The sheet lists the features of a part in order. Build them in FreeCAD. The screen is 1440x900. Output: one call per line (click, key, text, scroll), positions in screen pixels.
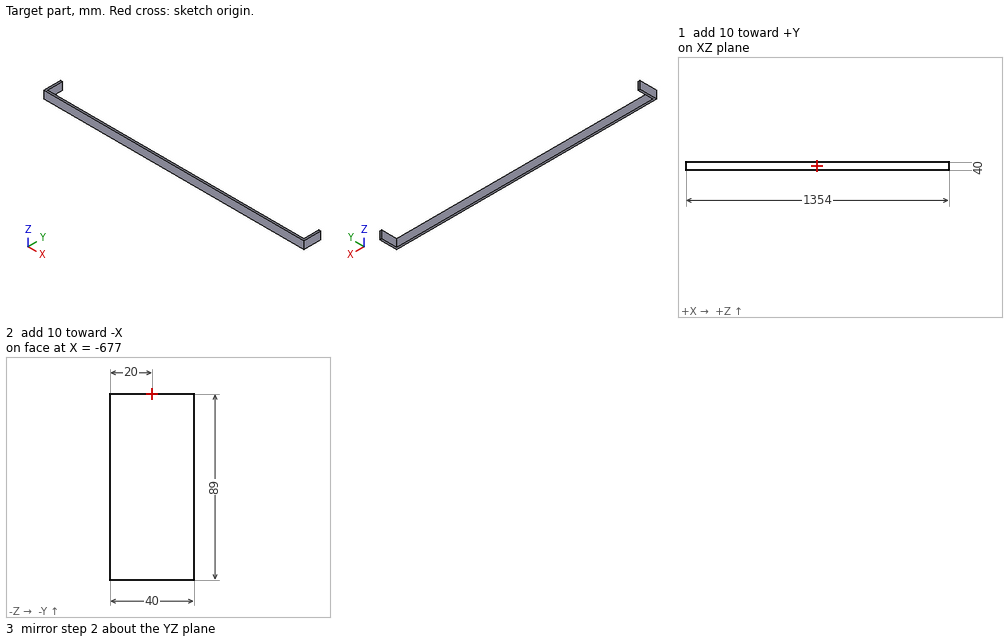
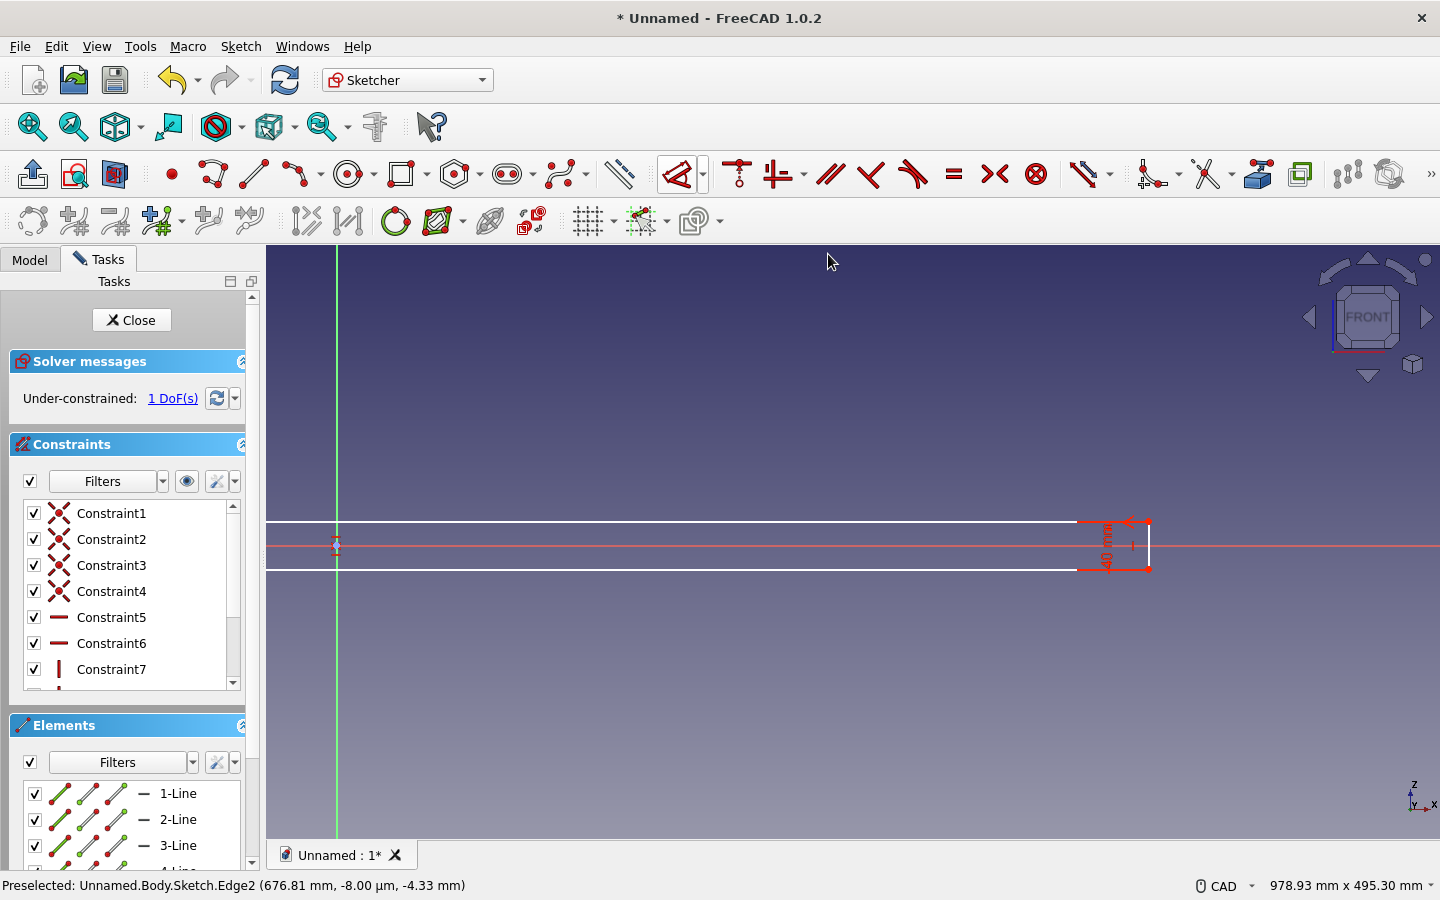
click(662, 570)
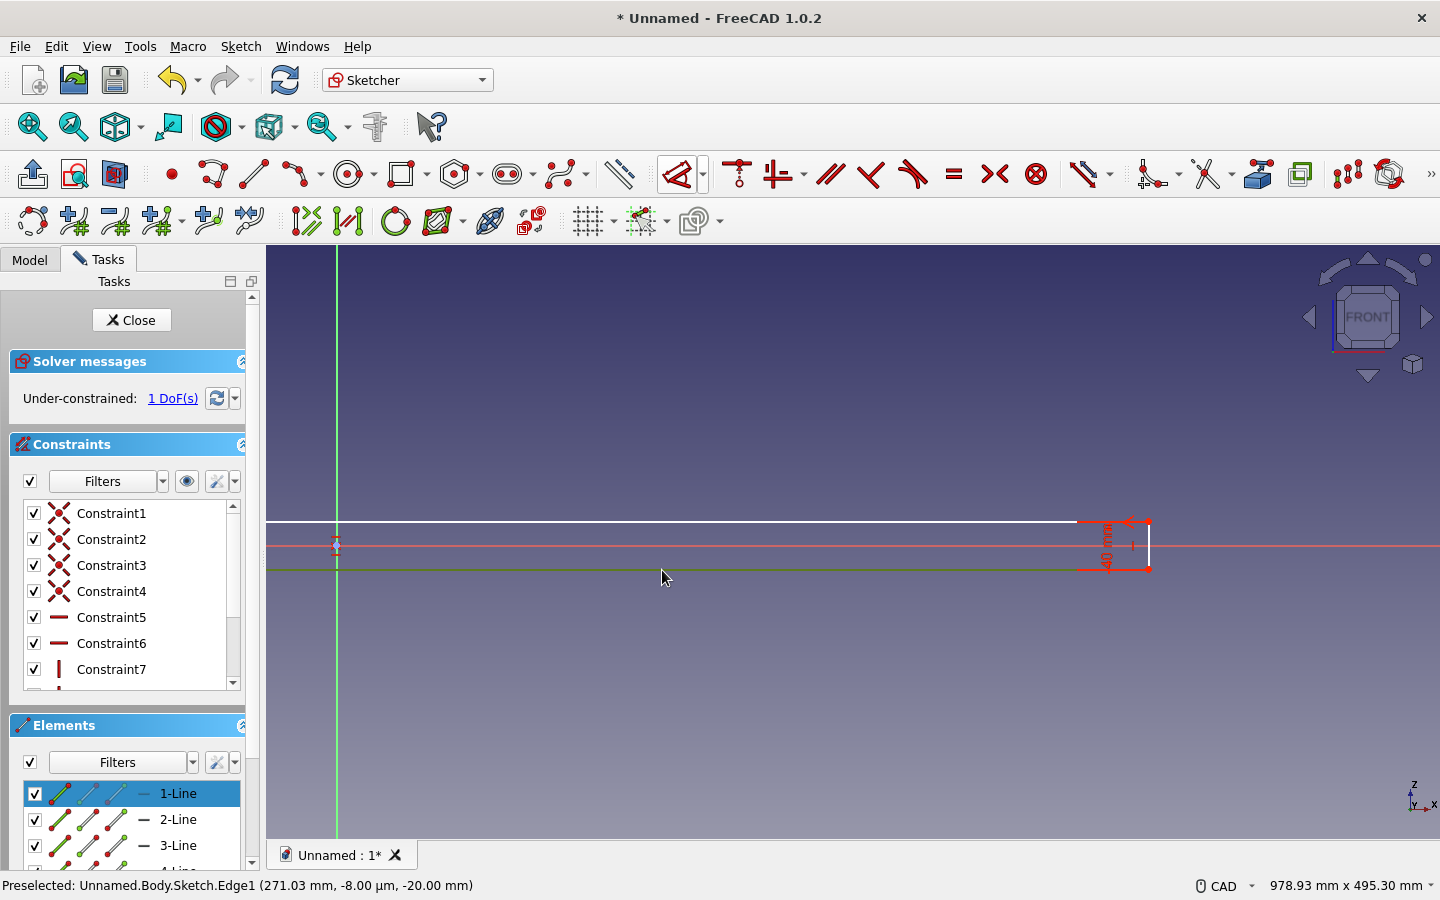
click(702, 174)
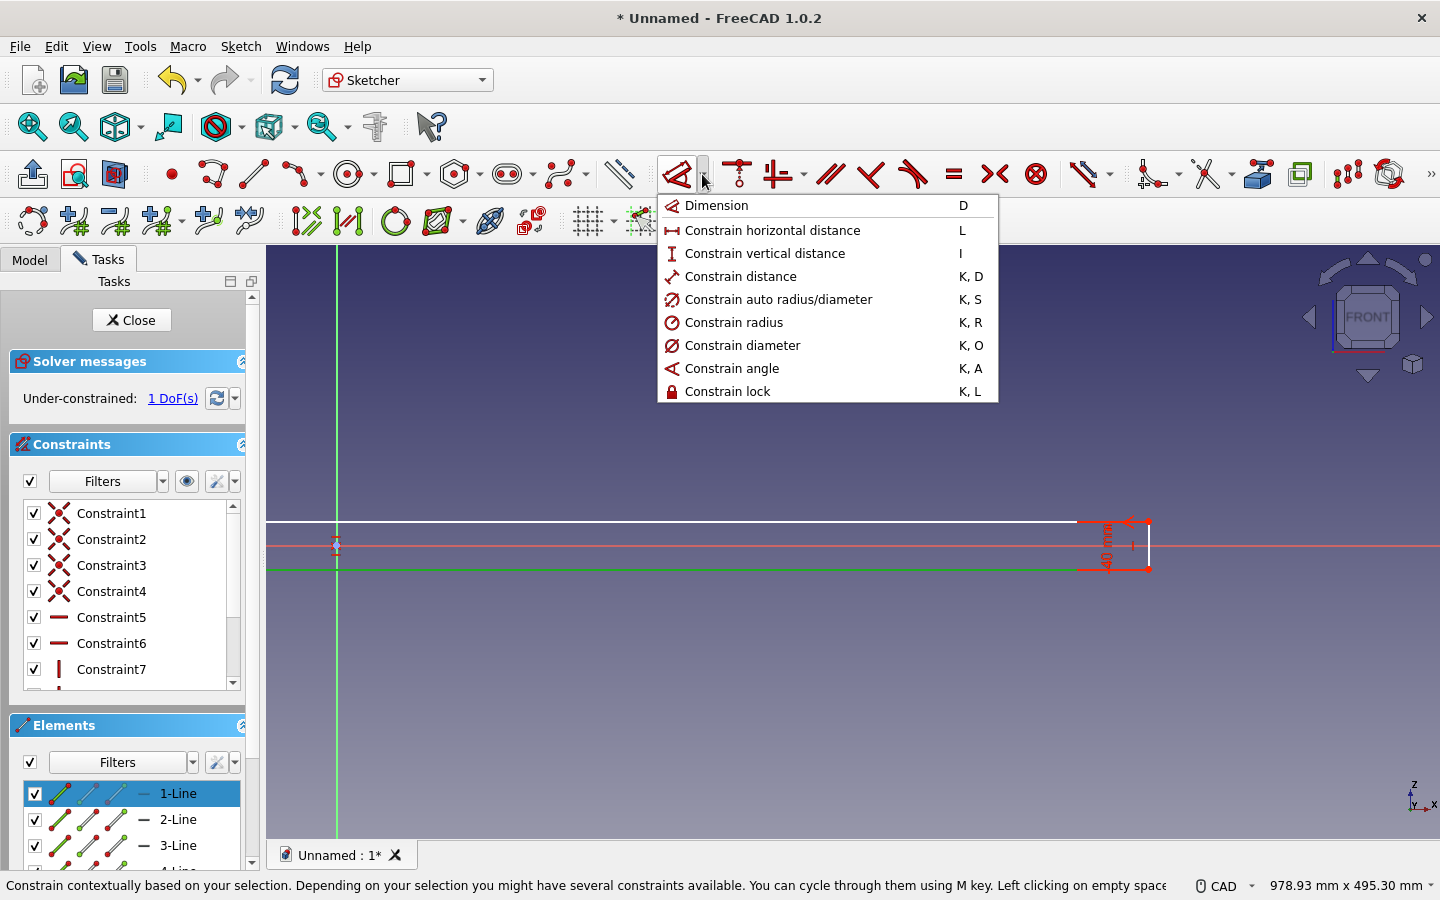
click(828, 230)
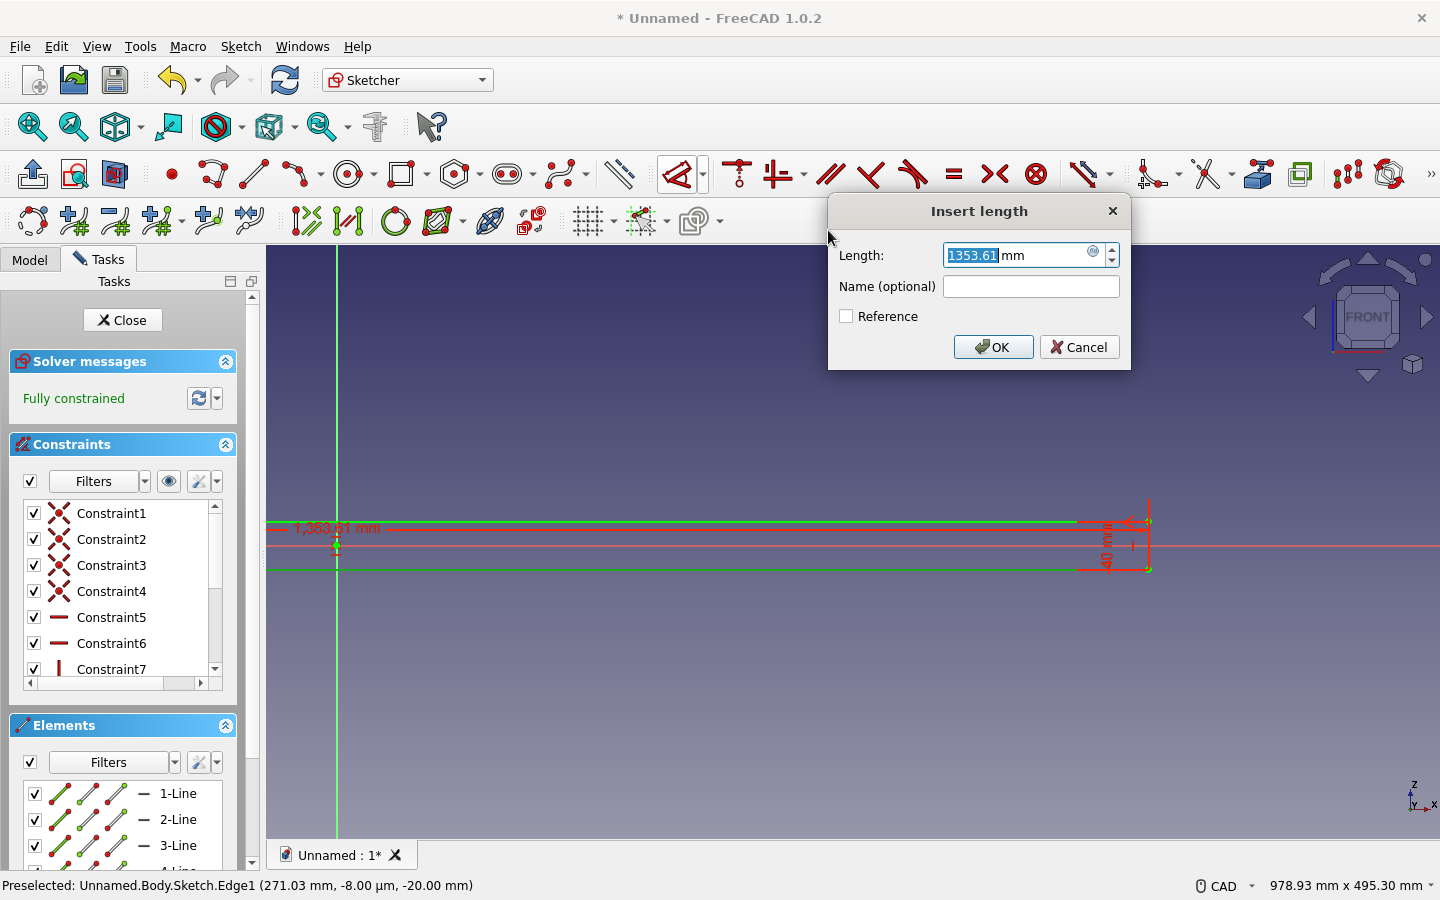
text(1354)
key(Return)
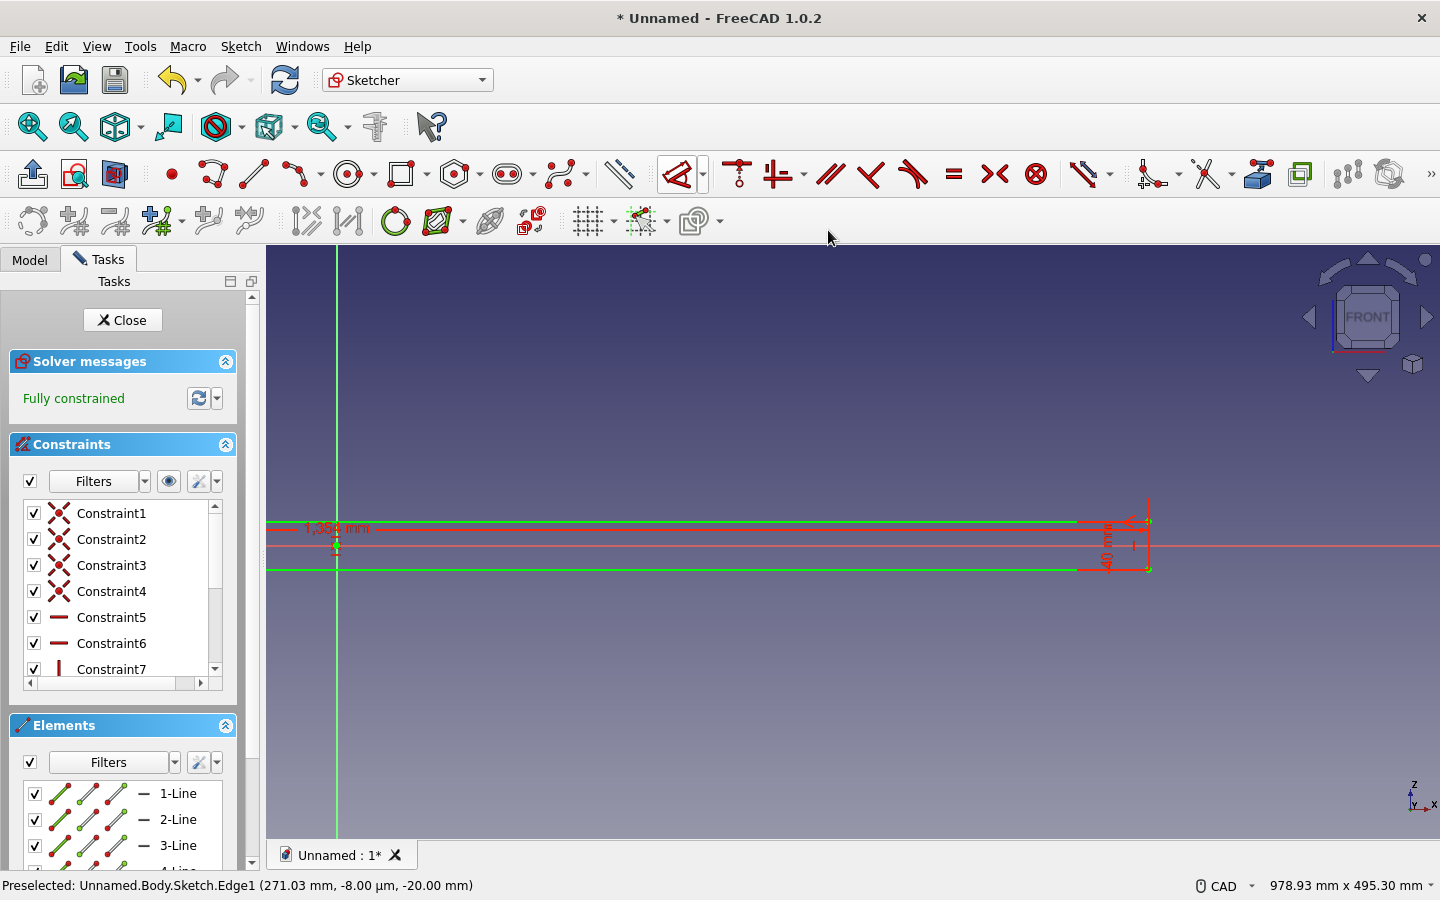
click(123, 320)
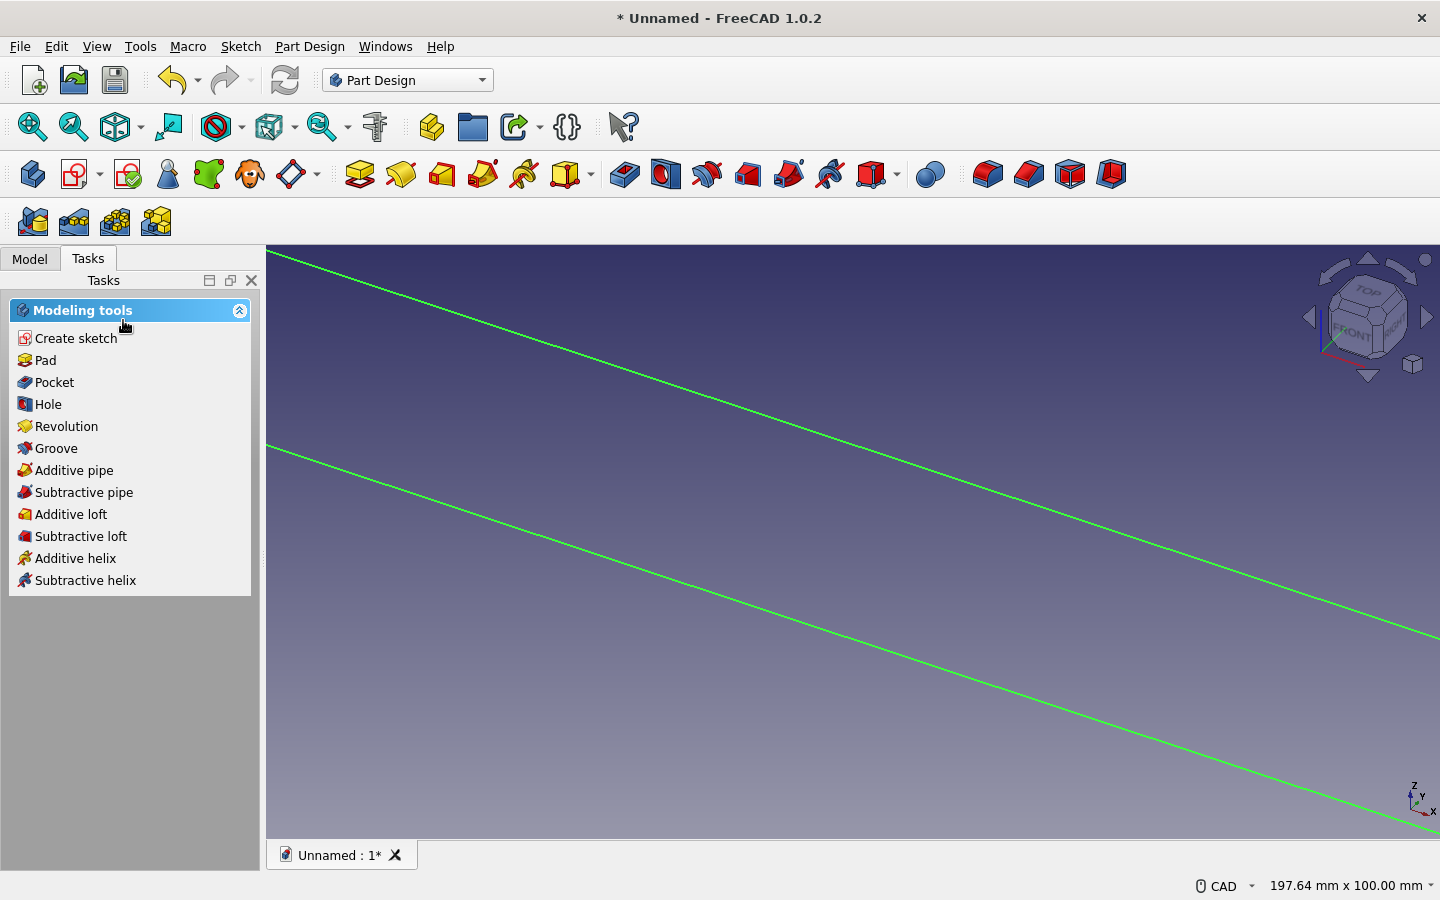
click(360, 174)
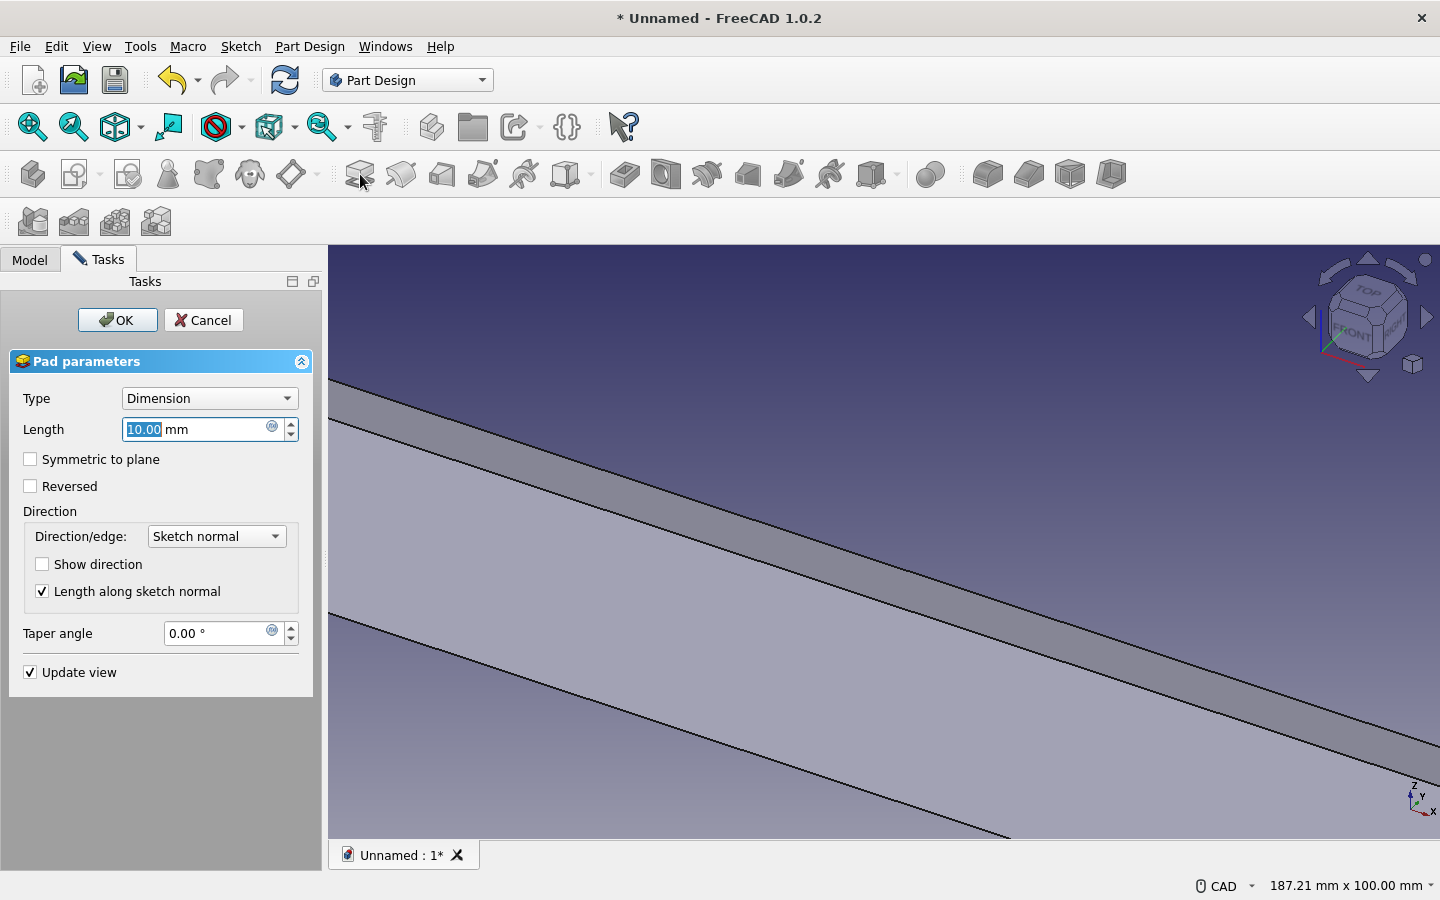
text(10)
key(Tab)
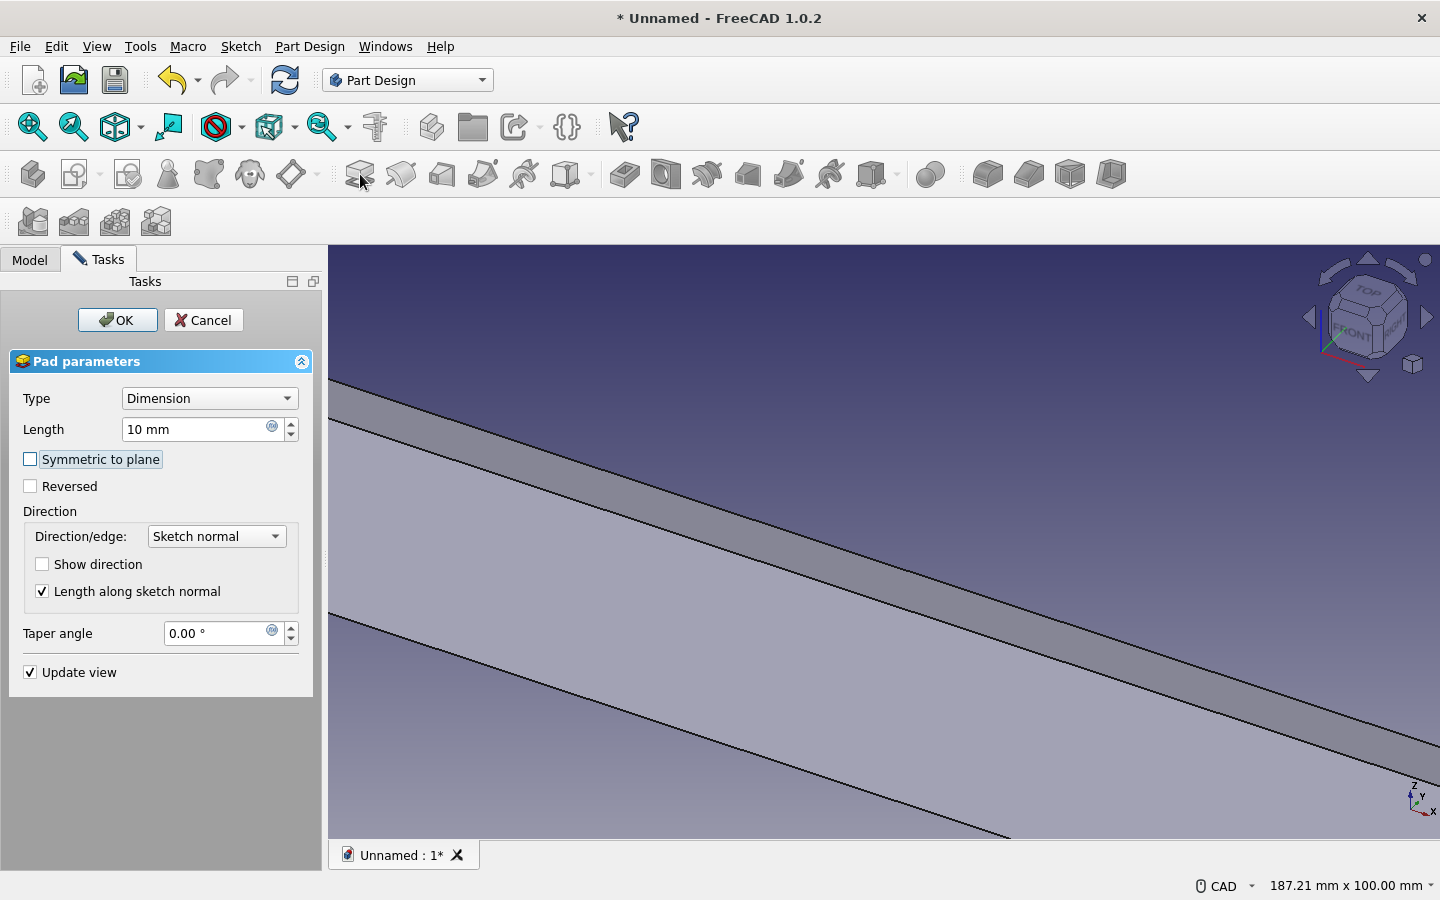
click(31, 486)